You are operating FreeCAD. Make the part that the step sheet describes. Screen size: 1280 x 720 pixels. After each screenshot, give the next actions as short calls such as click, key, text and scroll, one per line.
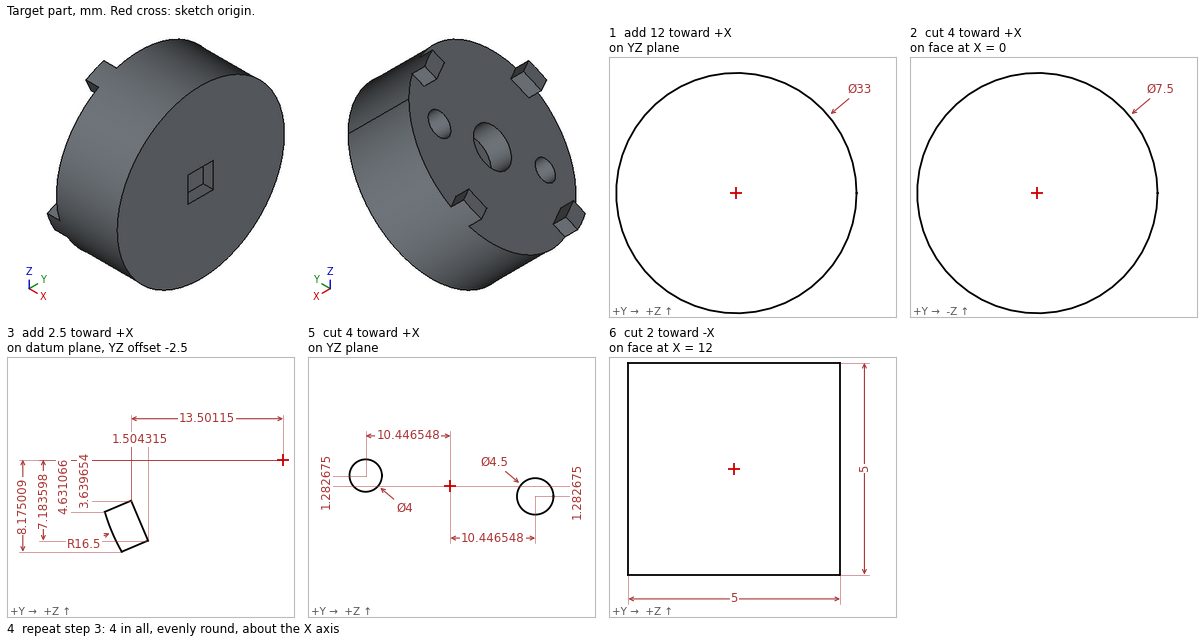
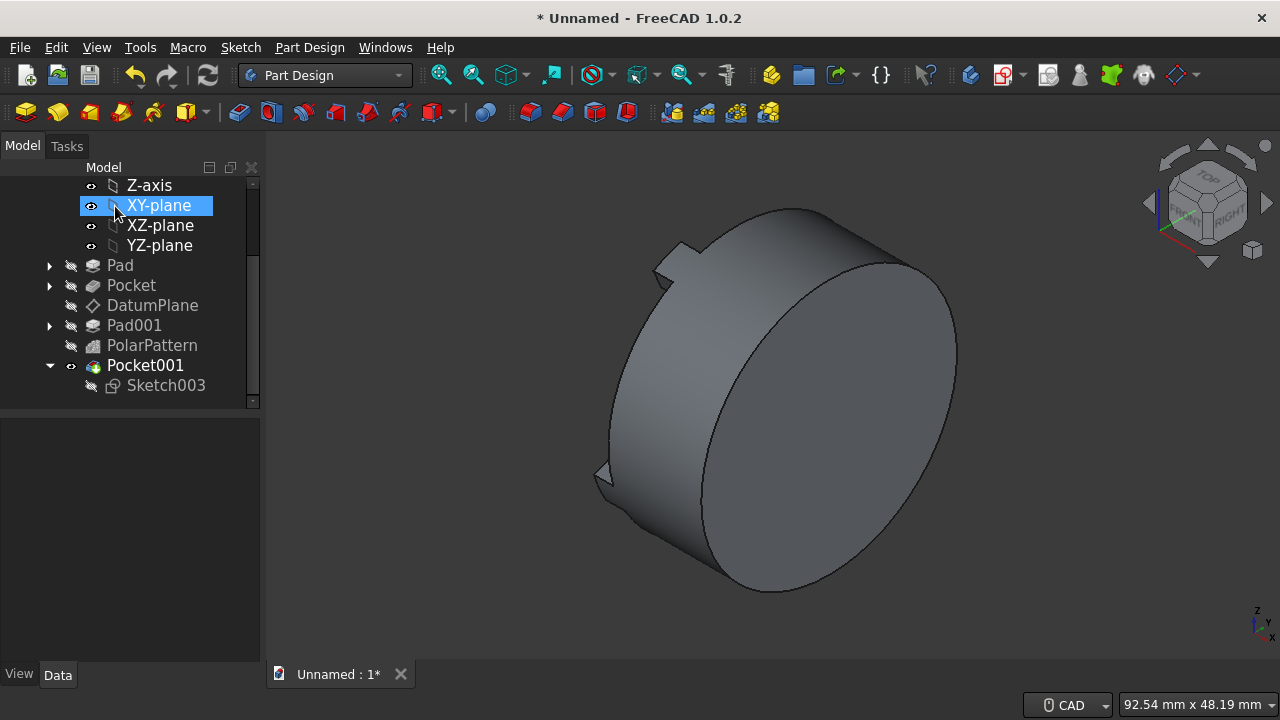
click(829, 426)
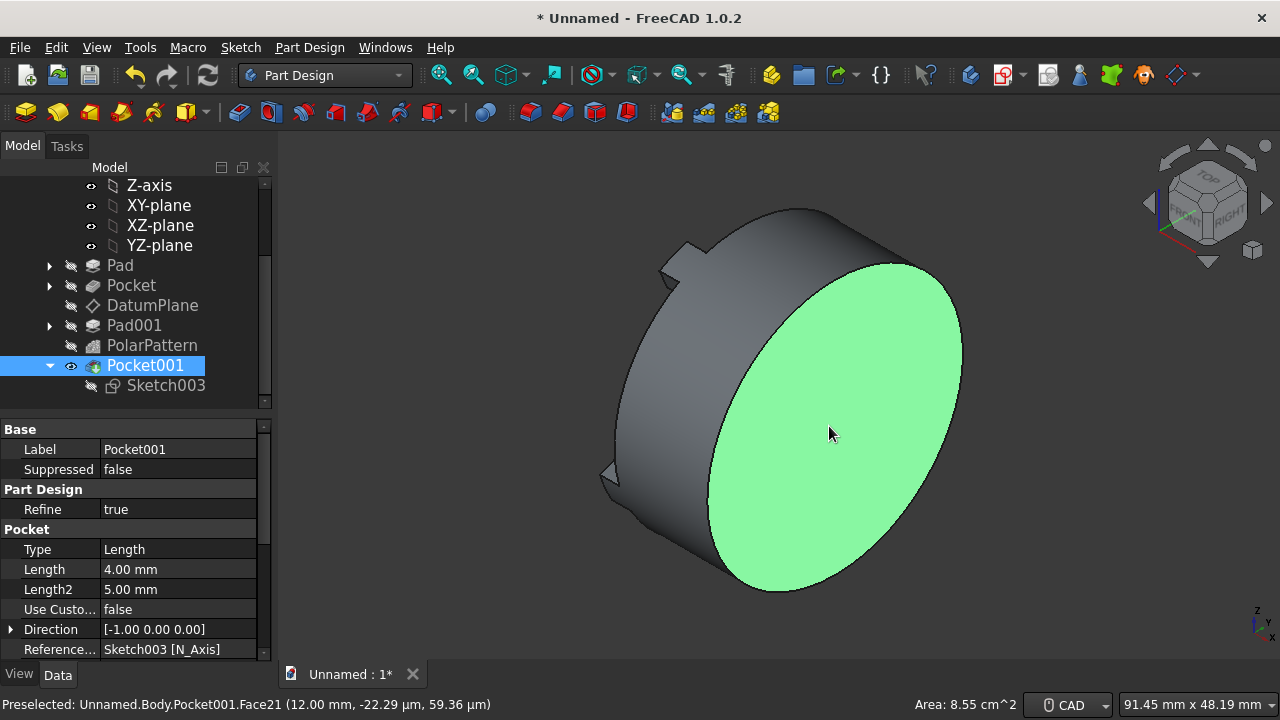
click(1004, 76)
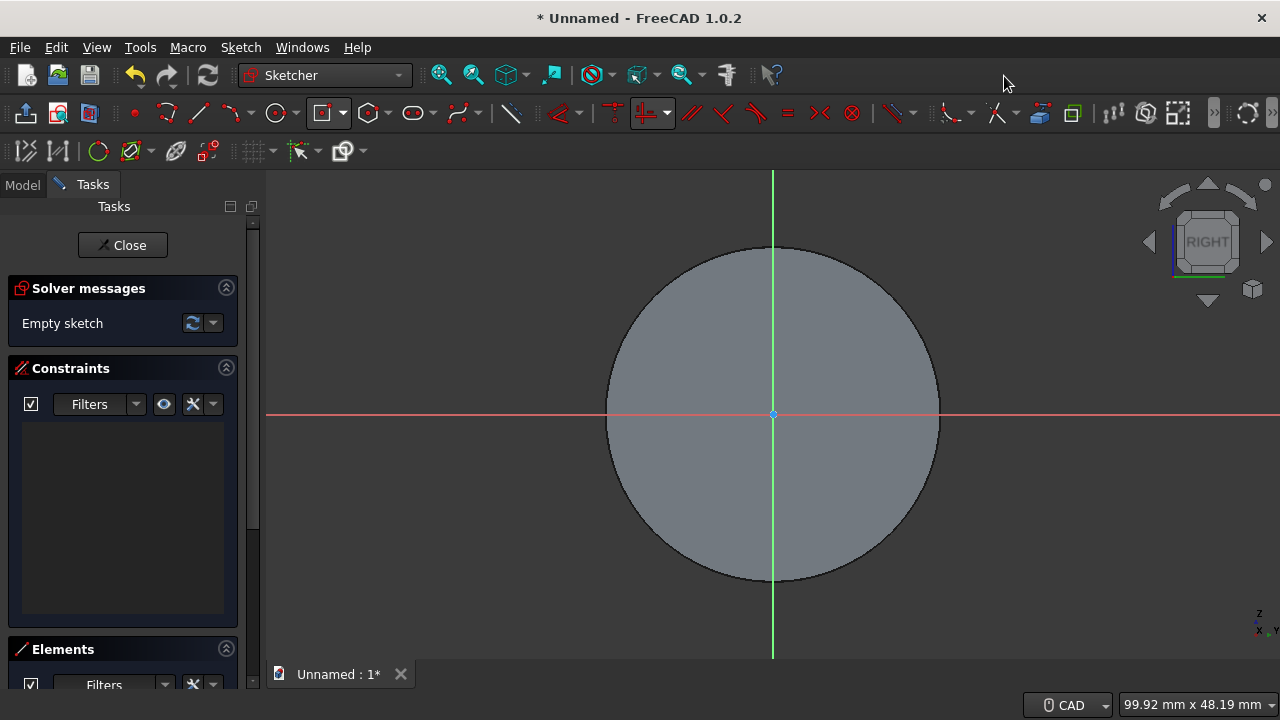
scroll(787, 415, up, 9)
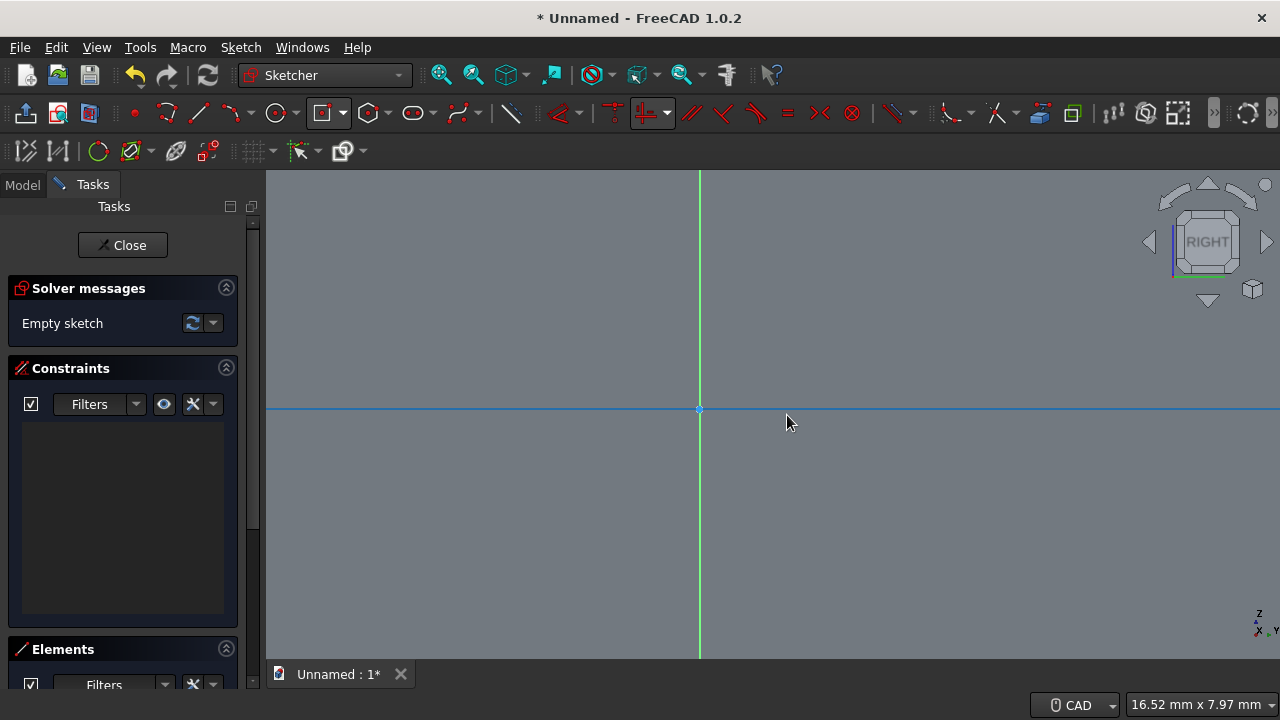
click(322, 114)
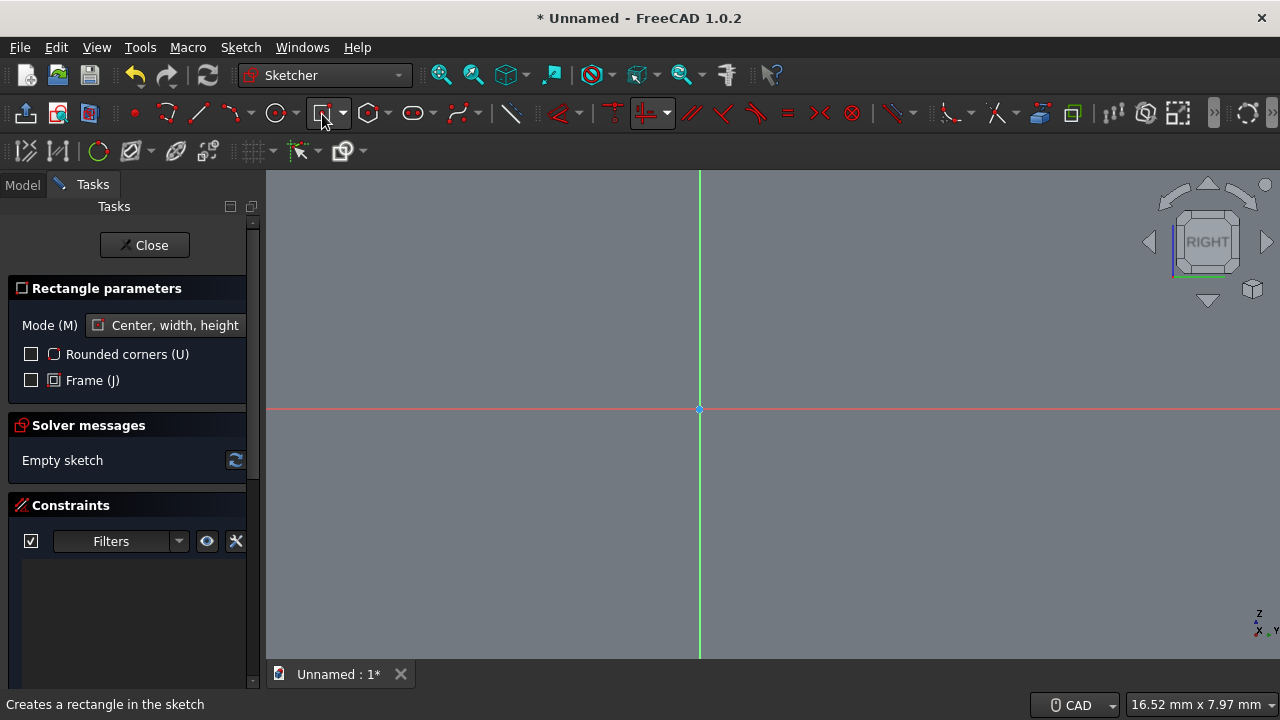
click(700, 409)
click(853, 256)
key(Escape)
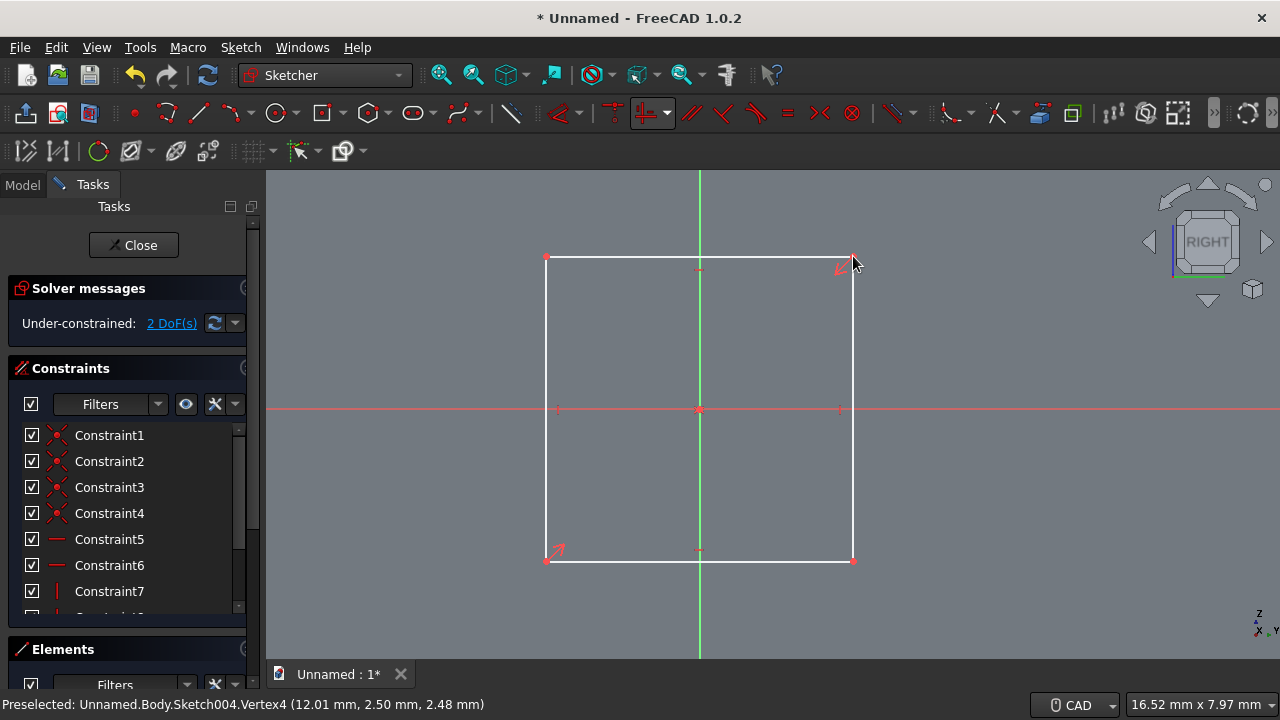
key(d)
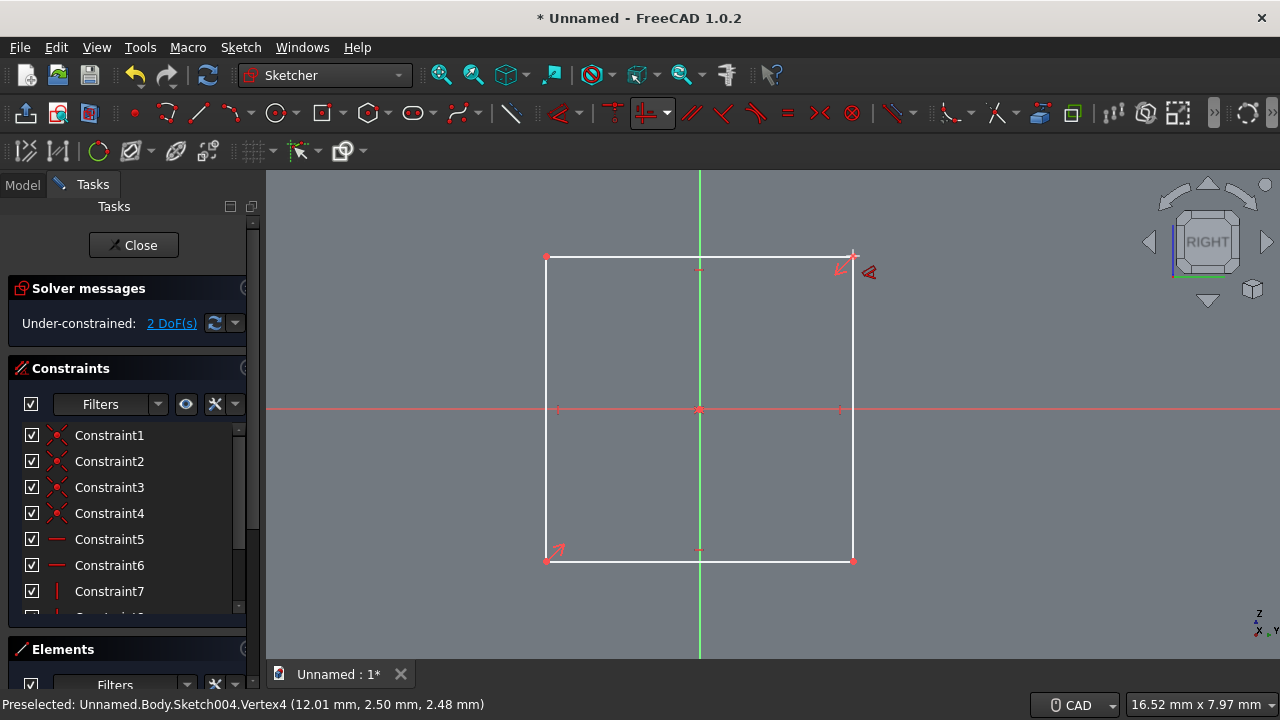
click(638, 562)
click(629, 596)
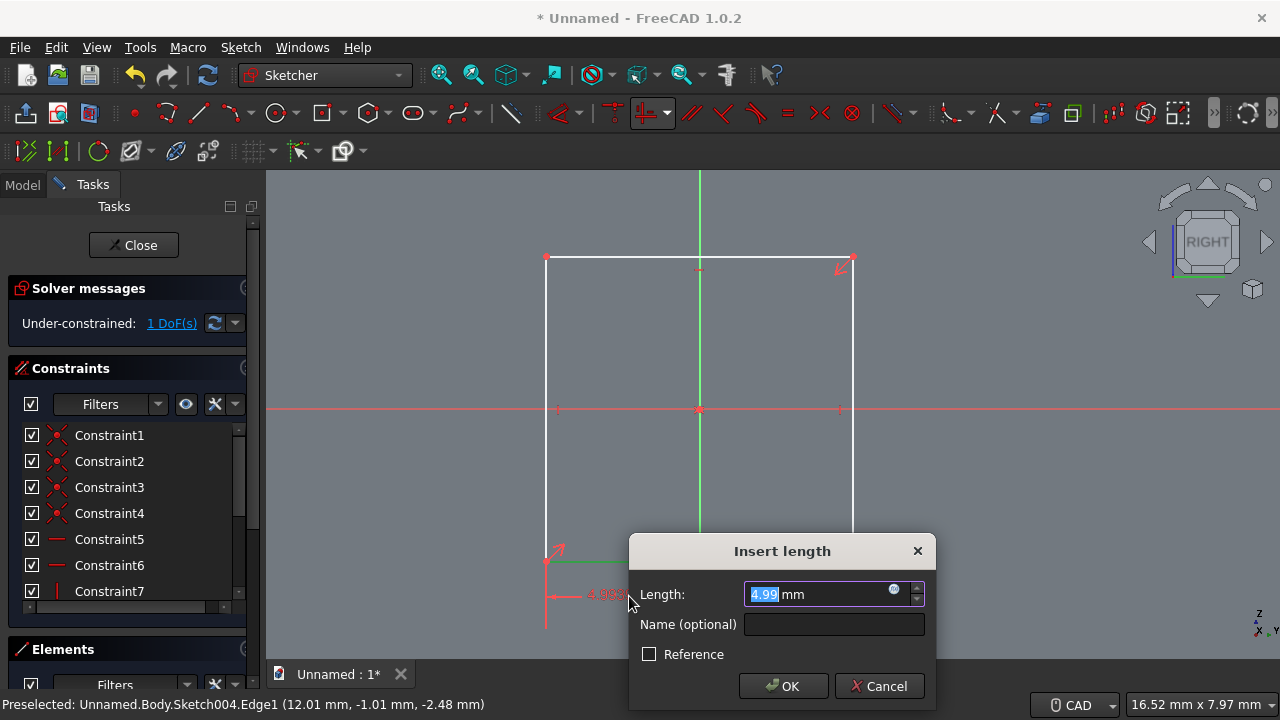
text(5)
key(Return)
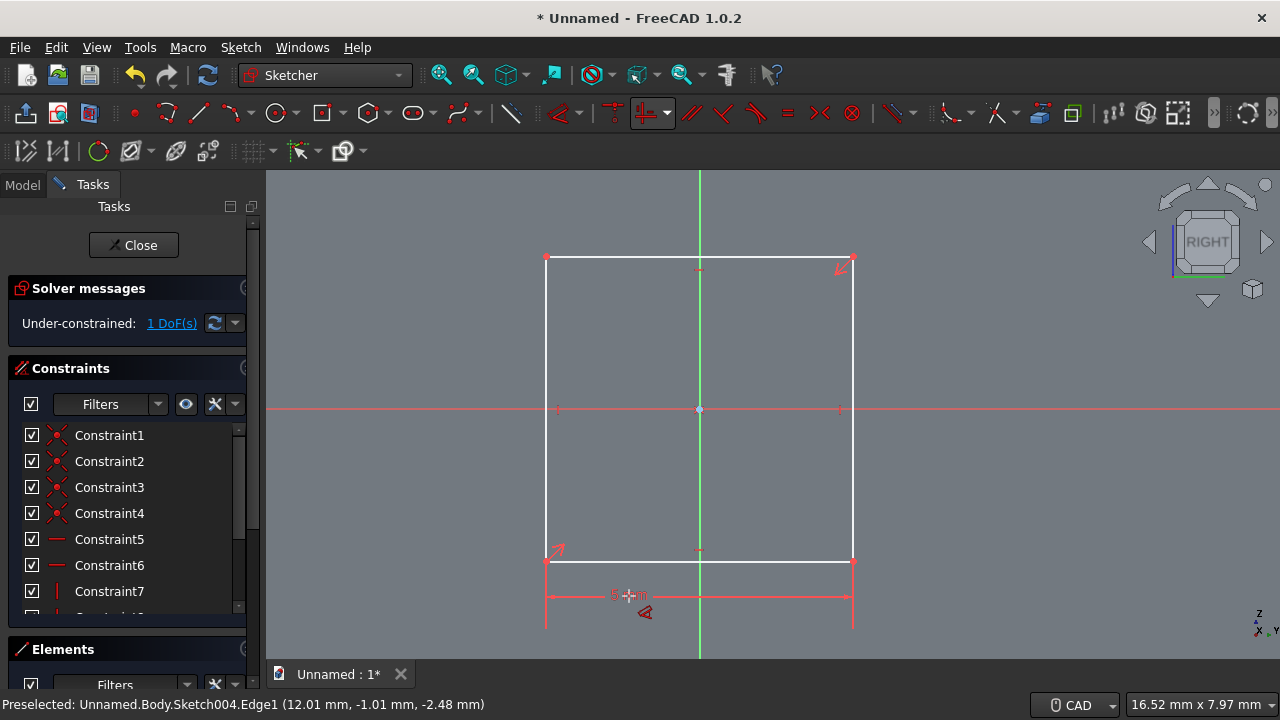
click(853, 470)
click(887, 339)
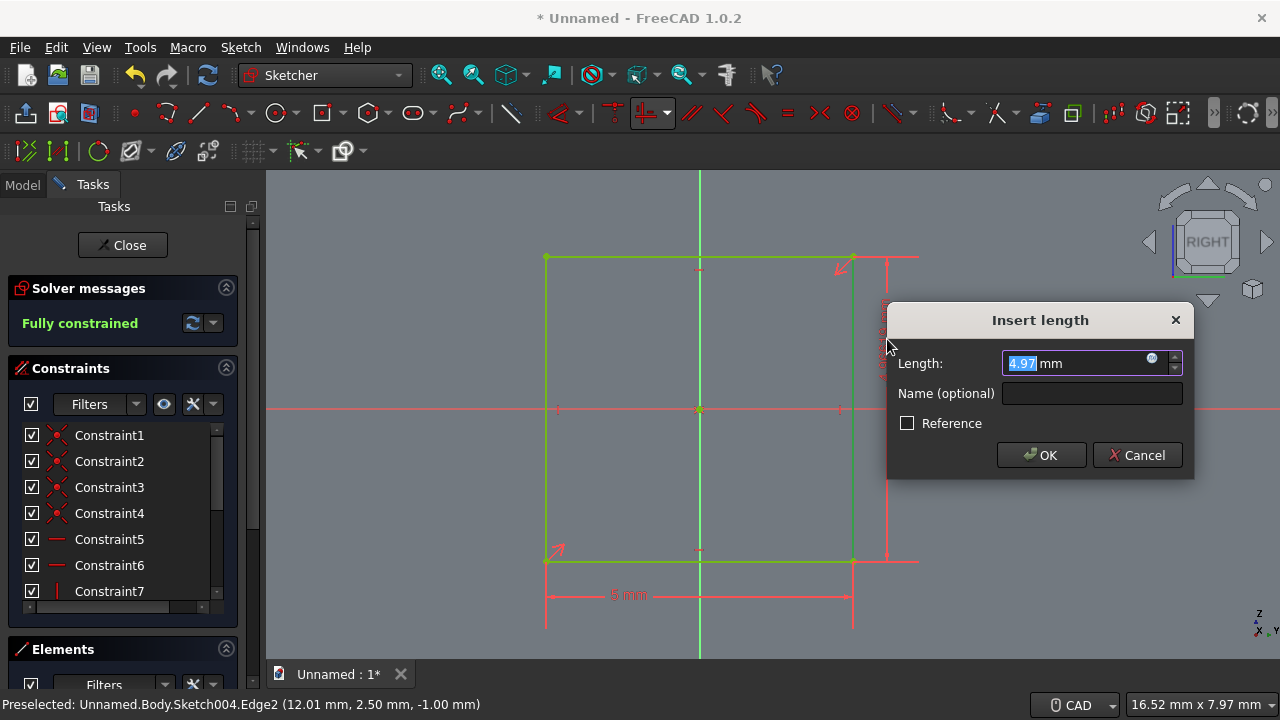
text(5)
key(Return)
key(Escape)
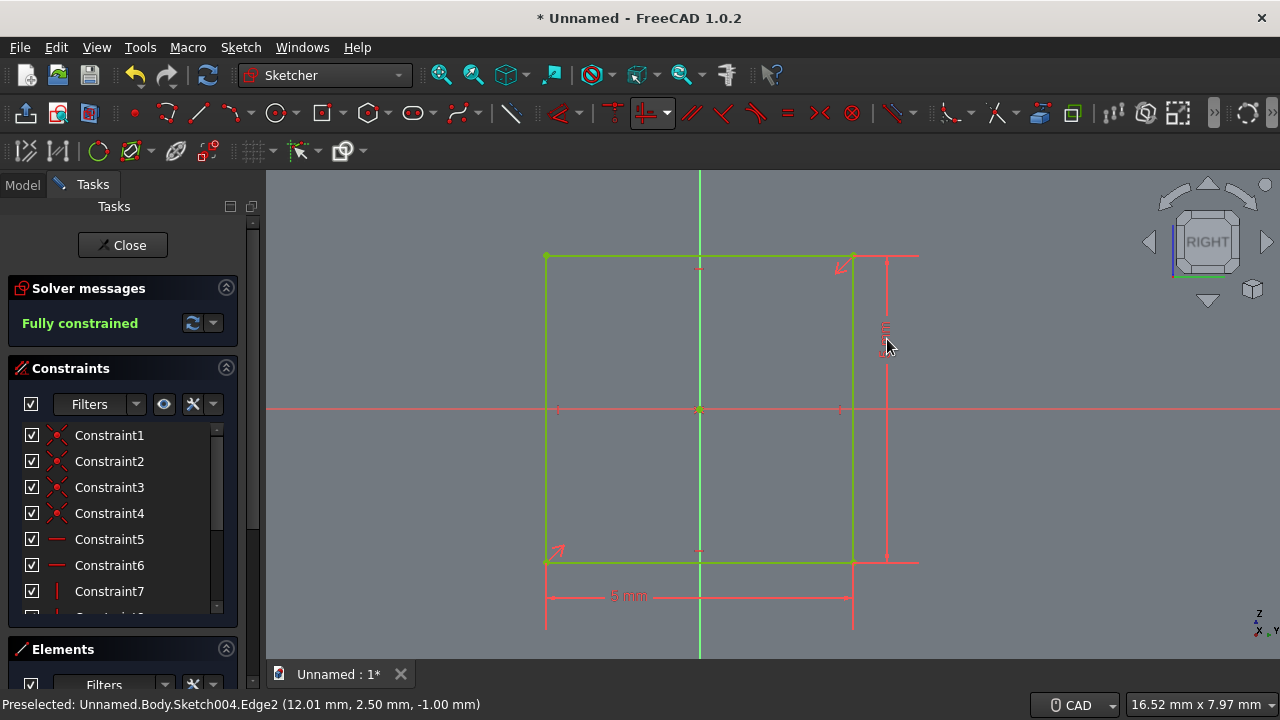
click(123, 245)